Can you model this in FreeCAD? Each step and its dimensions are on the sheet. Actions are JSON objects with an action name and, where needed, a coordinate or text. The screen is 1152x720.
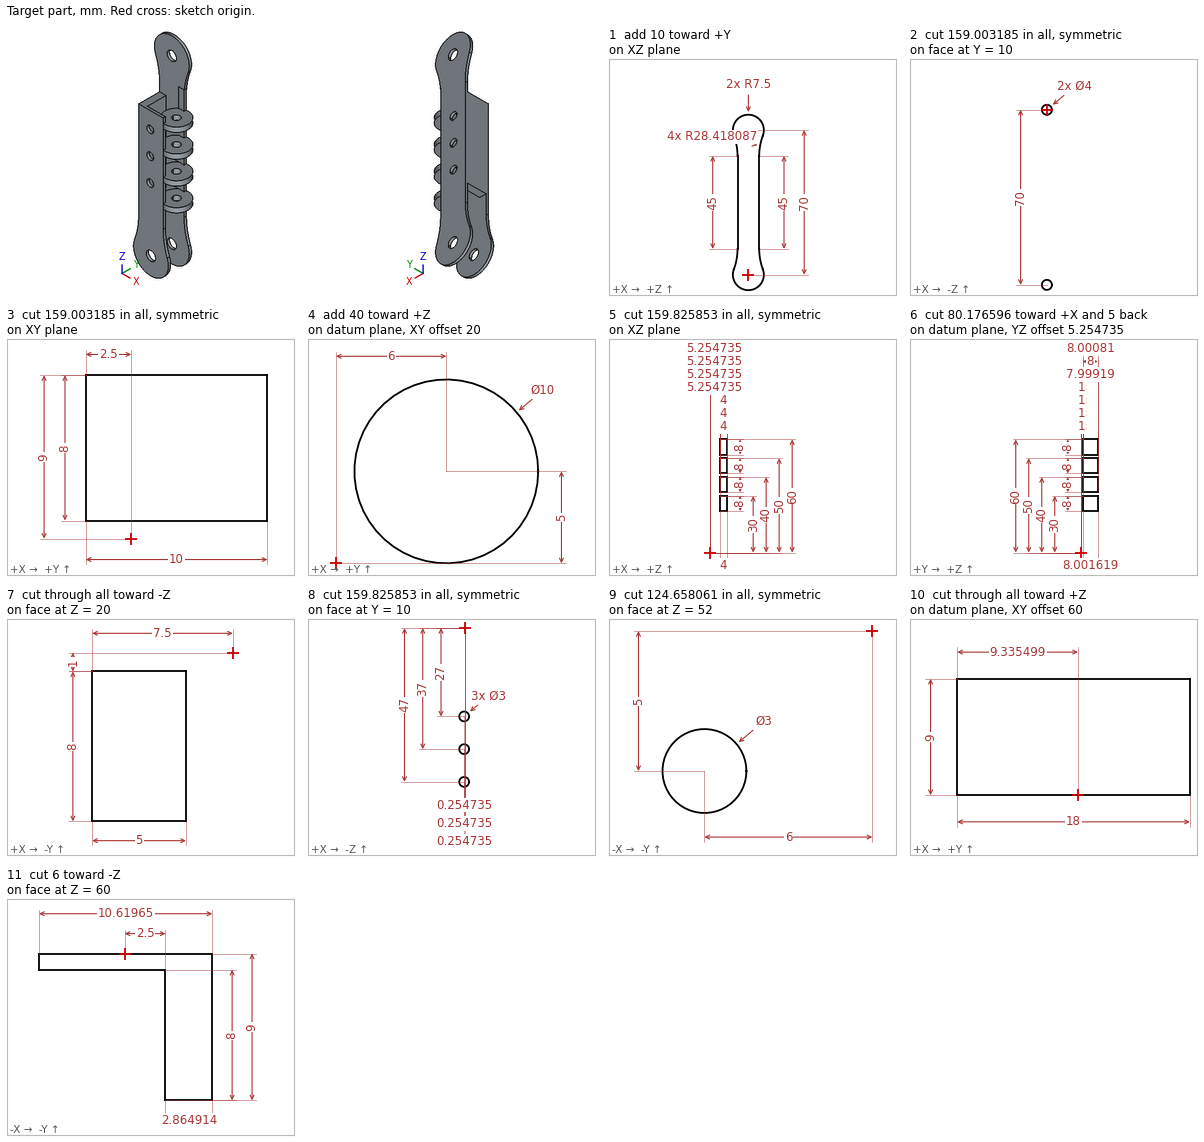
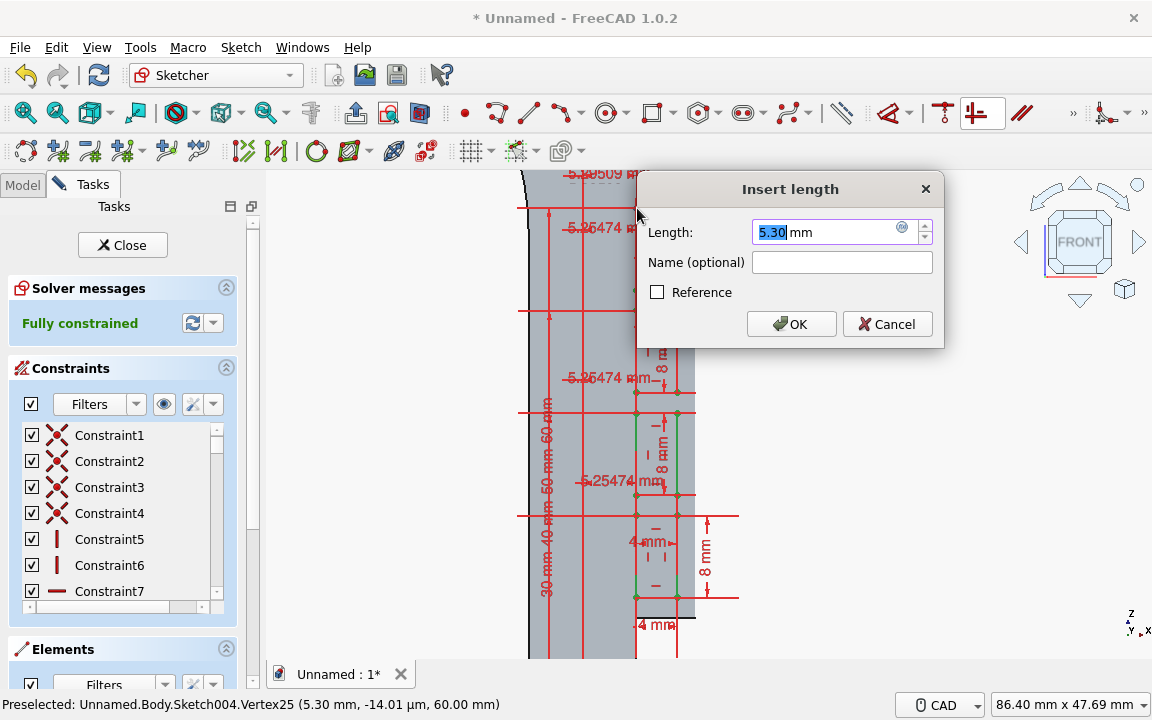
{"action": "type", "text": "5.254735"}
{"action": "key", "text": "Return"}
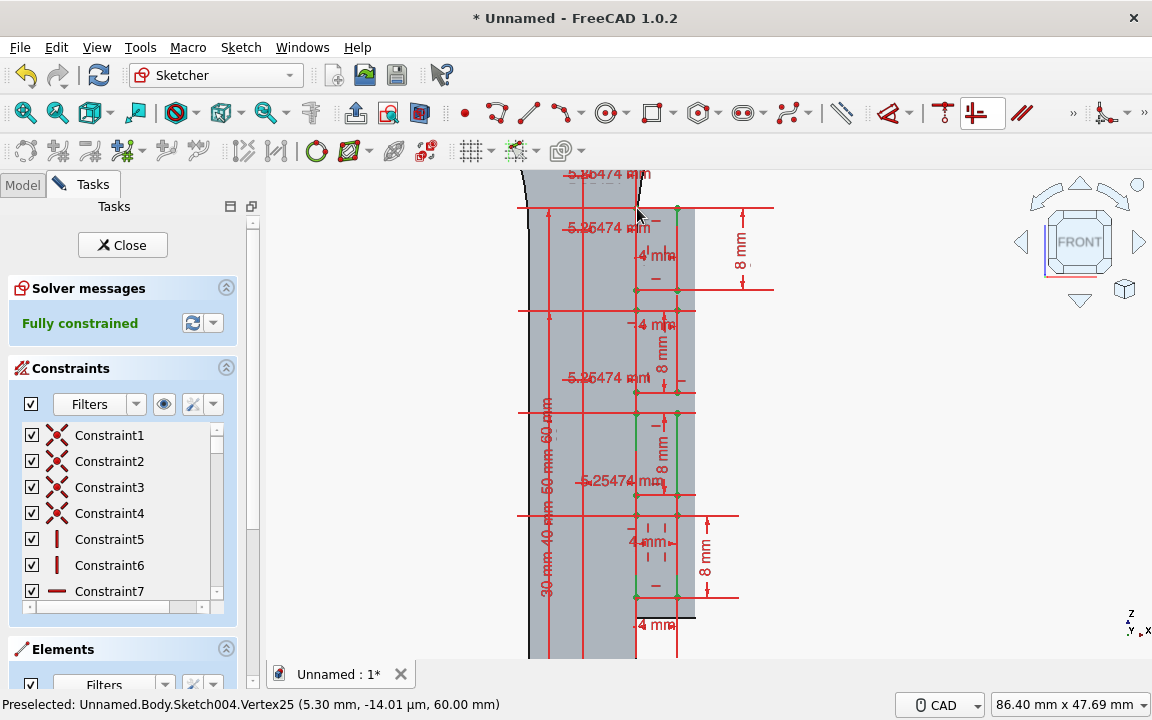
{"action": "left_click", "coordinate": [123, 245]}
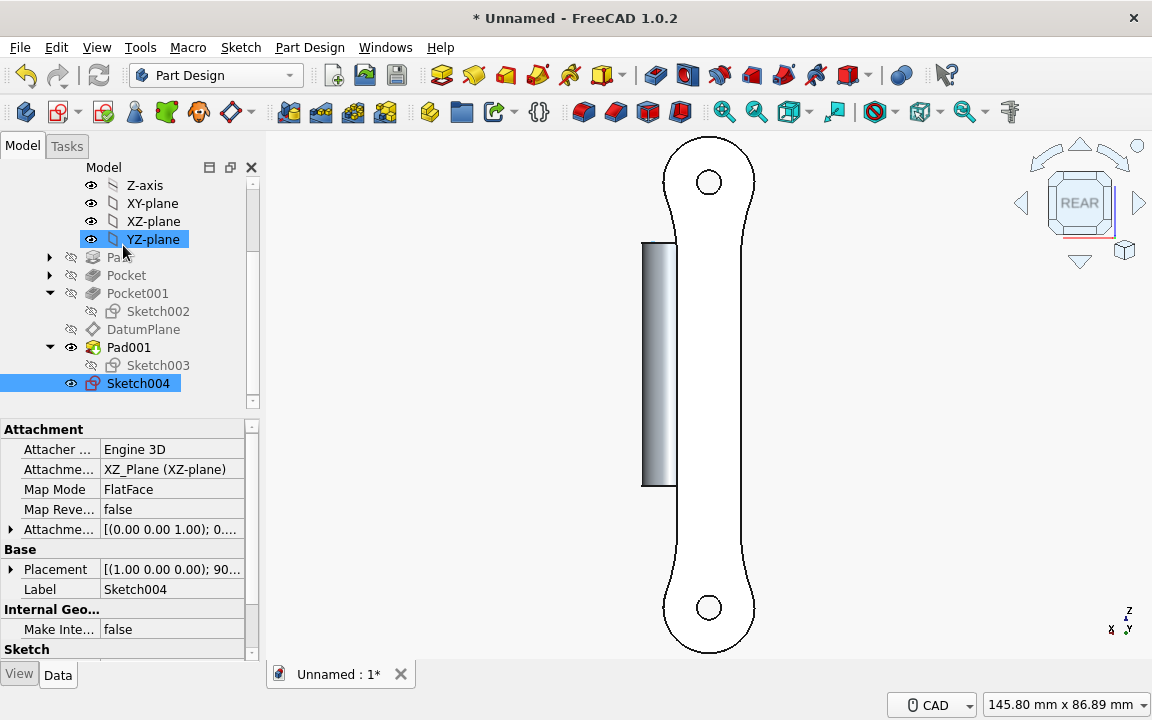
{"action": "left_click", "coordinate": [656, 76]}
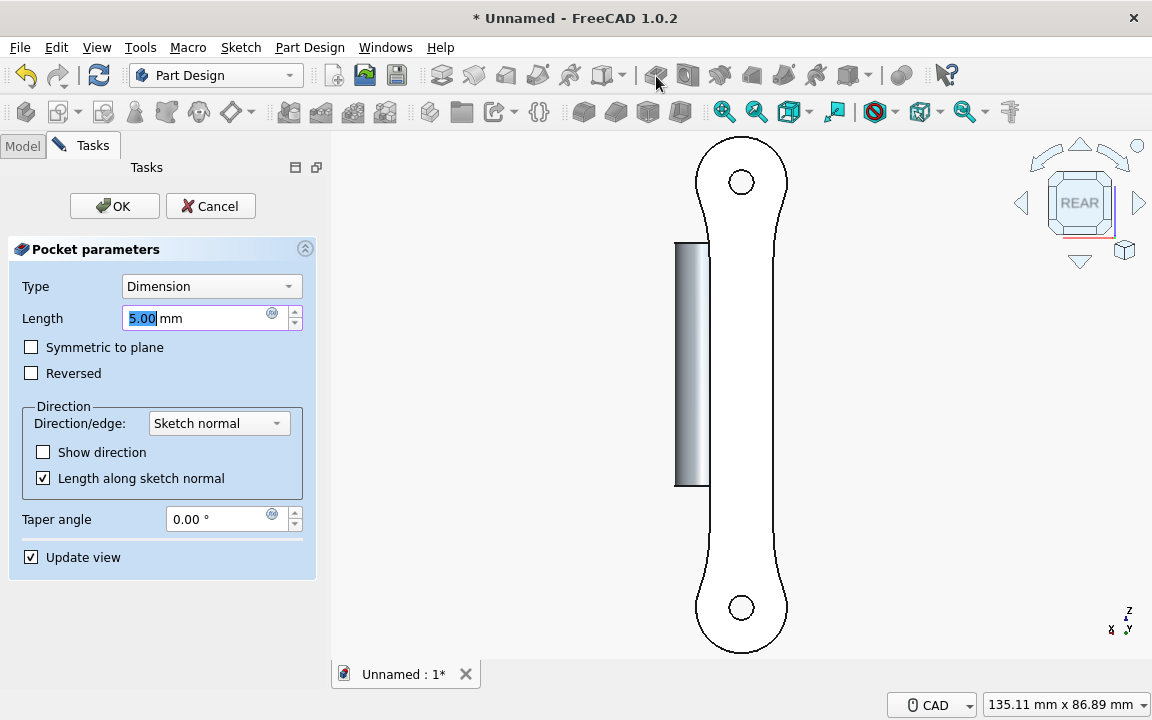
{"action": "type", "text": "159.825853"}
{"action": "key", "text": "Tab"}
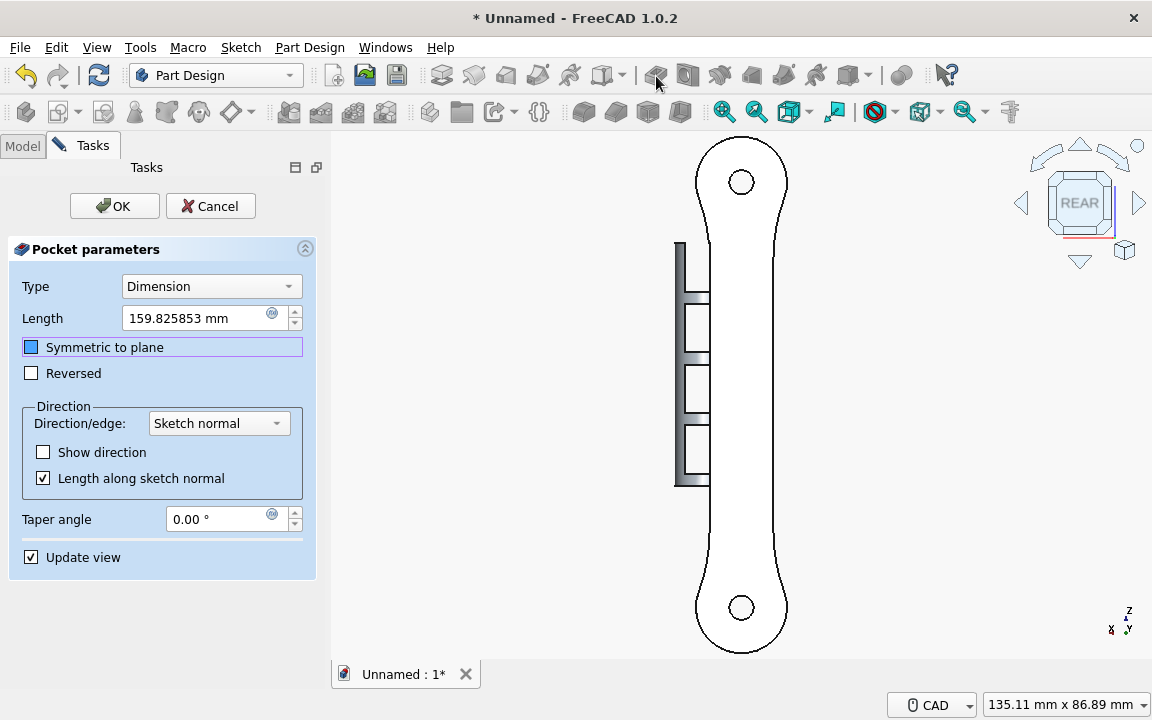
{"action": "left_click", "coordinate": [30, 347]}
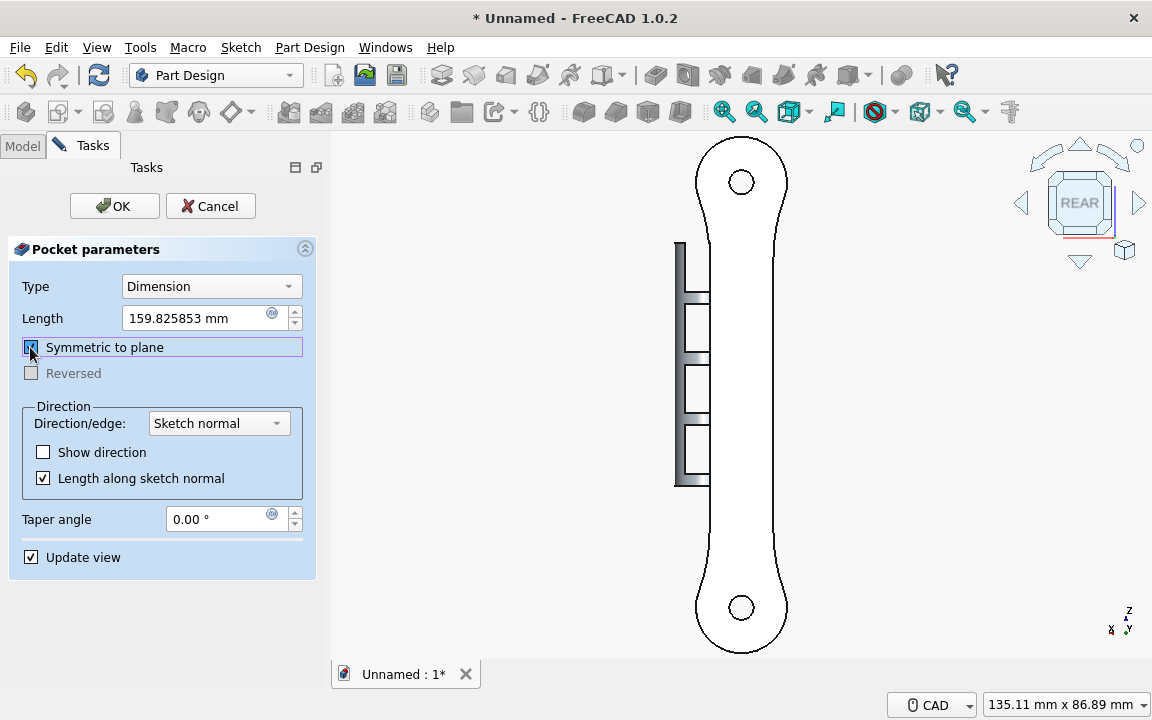
{"action": "left_click", "coordinate": [115, 206]}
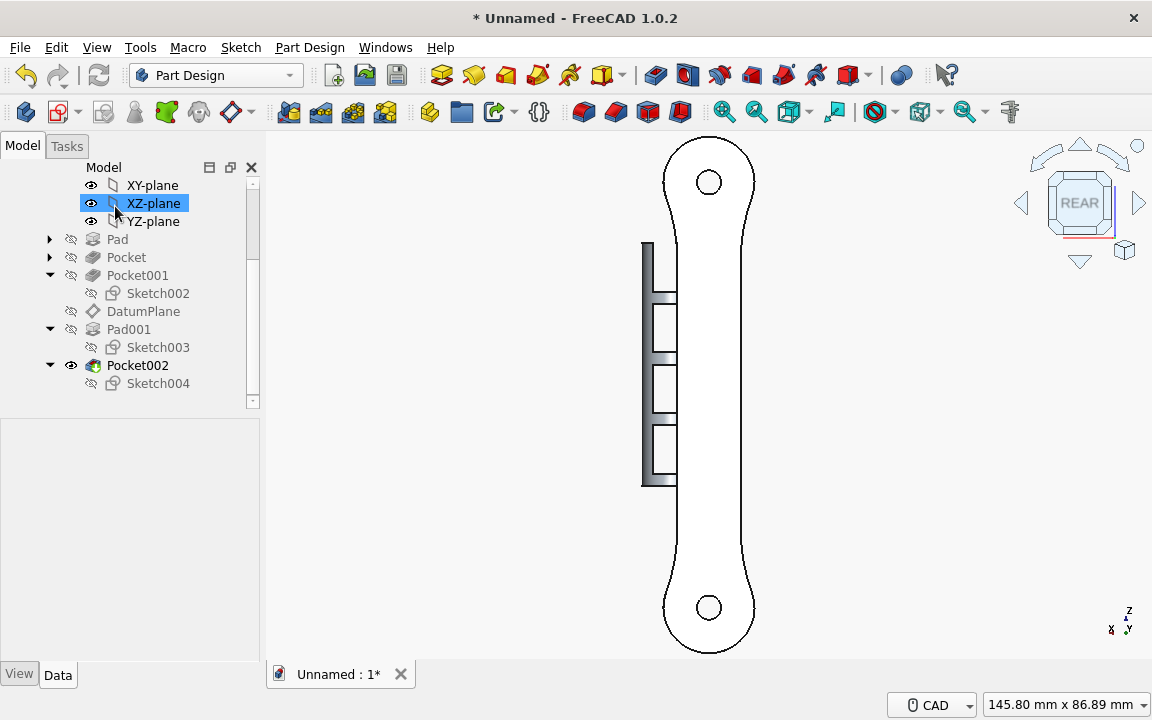
{"action": "scroll", "coordinate": [160, 289], "scroll_direction": "down", "scroll_amount": 3}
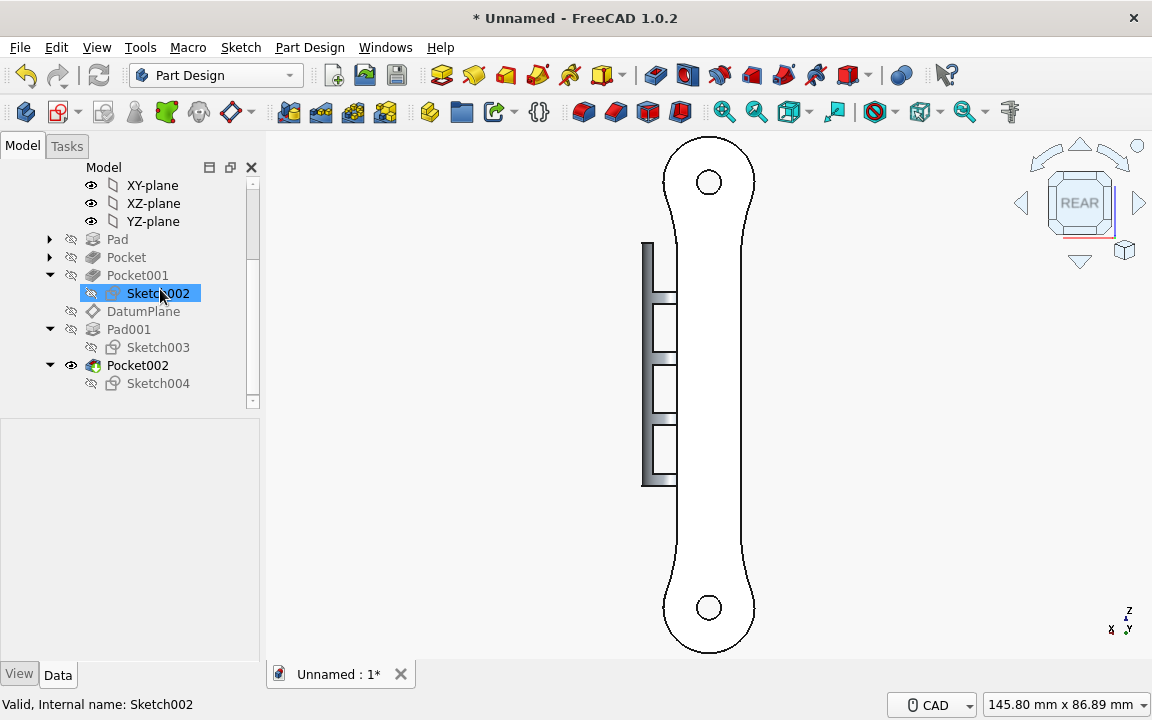
{"action": "scroll", "coordinate": [160, 289], "scroll_direction": "up", "scroll_amount": 15}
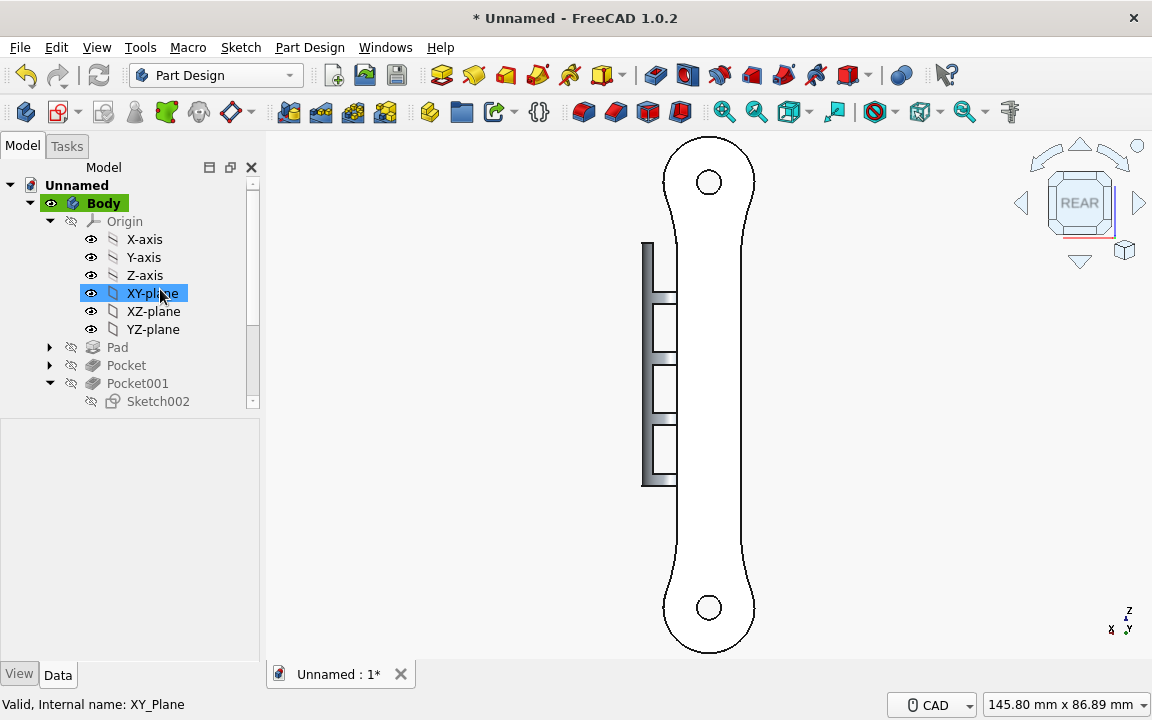
{"action": "left_click", "coordinate": [136, 329]}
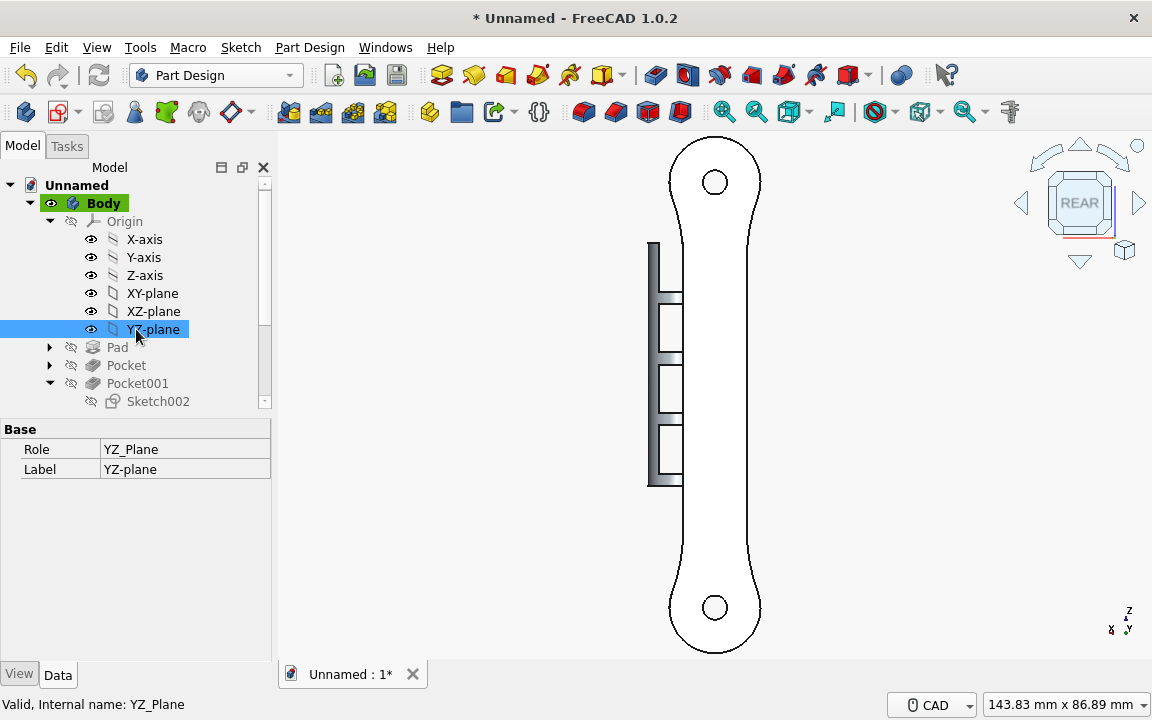
{"action": "left_click", "coordinate": [232, 112]}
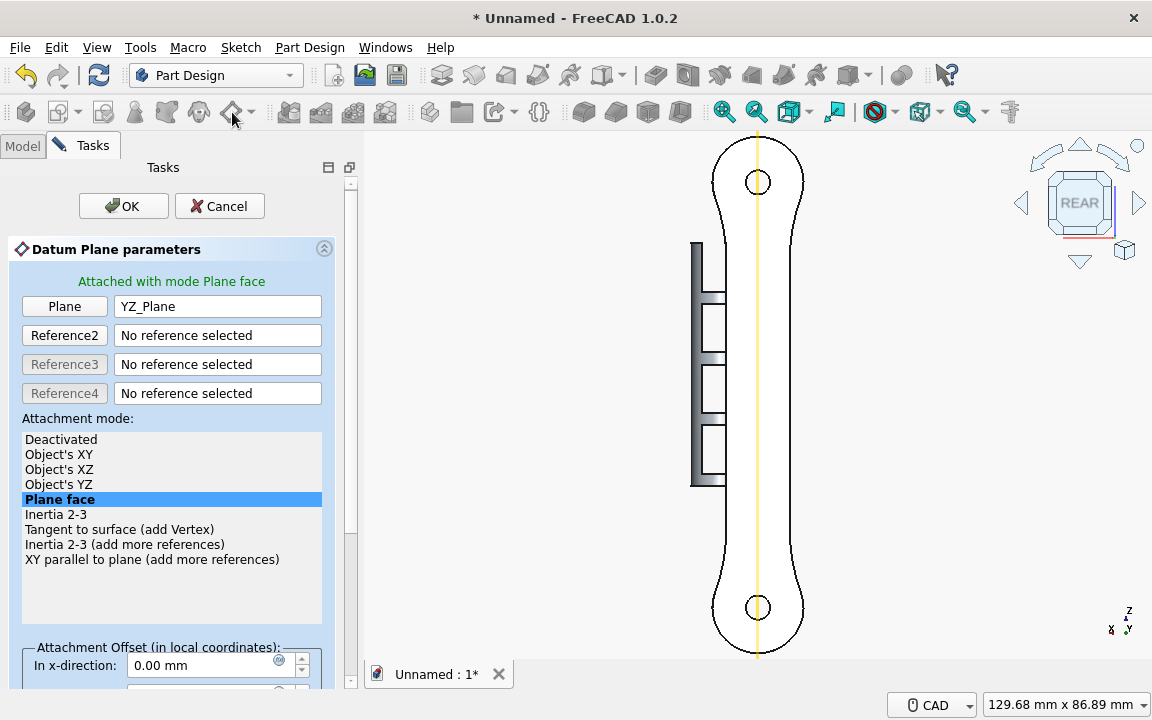
{"action": "scroll", "coordinate": [351, 432], "scroll_direction": "down", "scroll_amount": 2}